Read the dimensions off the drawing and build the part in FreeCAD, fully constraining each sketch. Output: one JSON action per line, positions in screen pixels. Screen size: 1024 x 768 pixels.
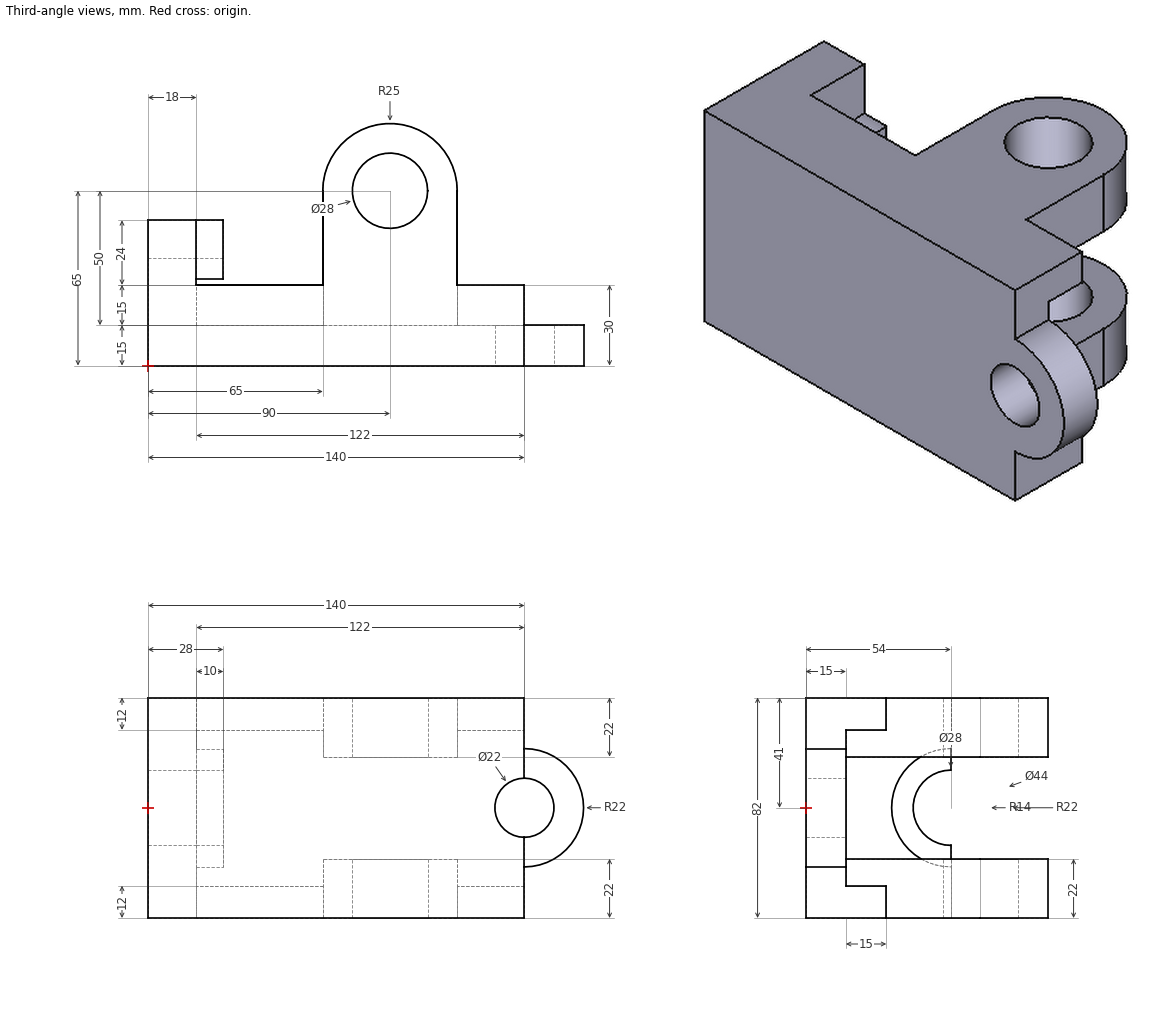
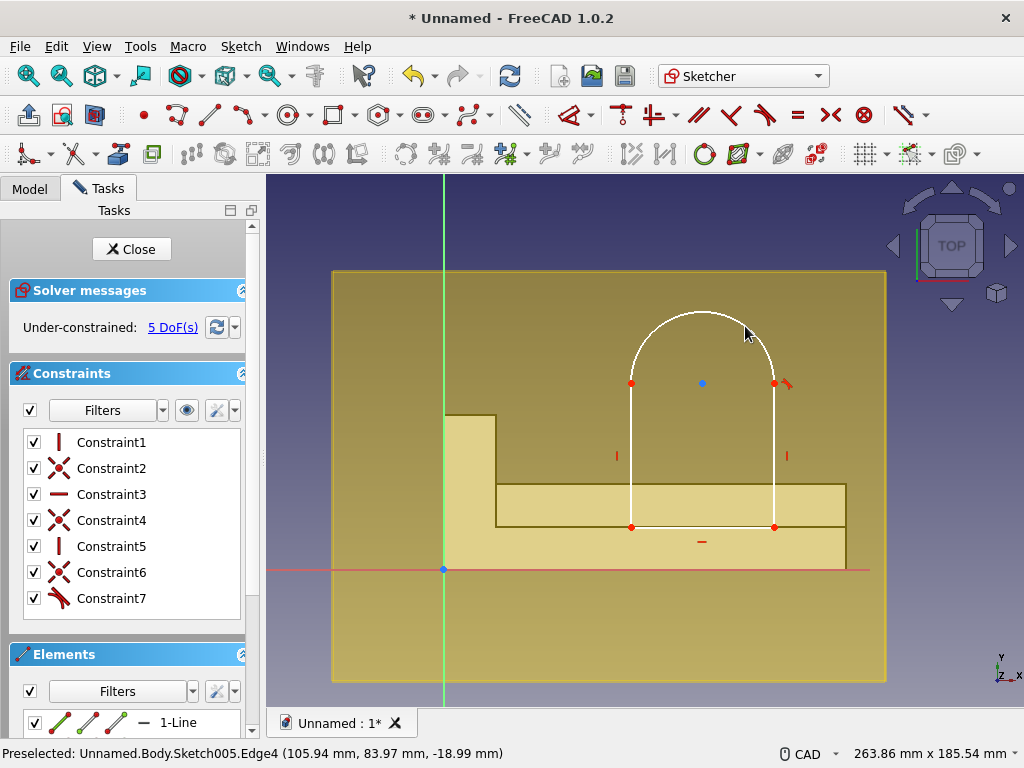
{"action": "left_click", "coordinate": [631, 485]}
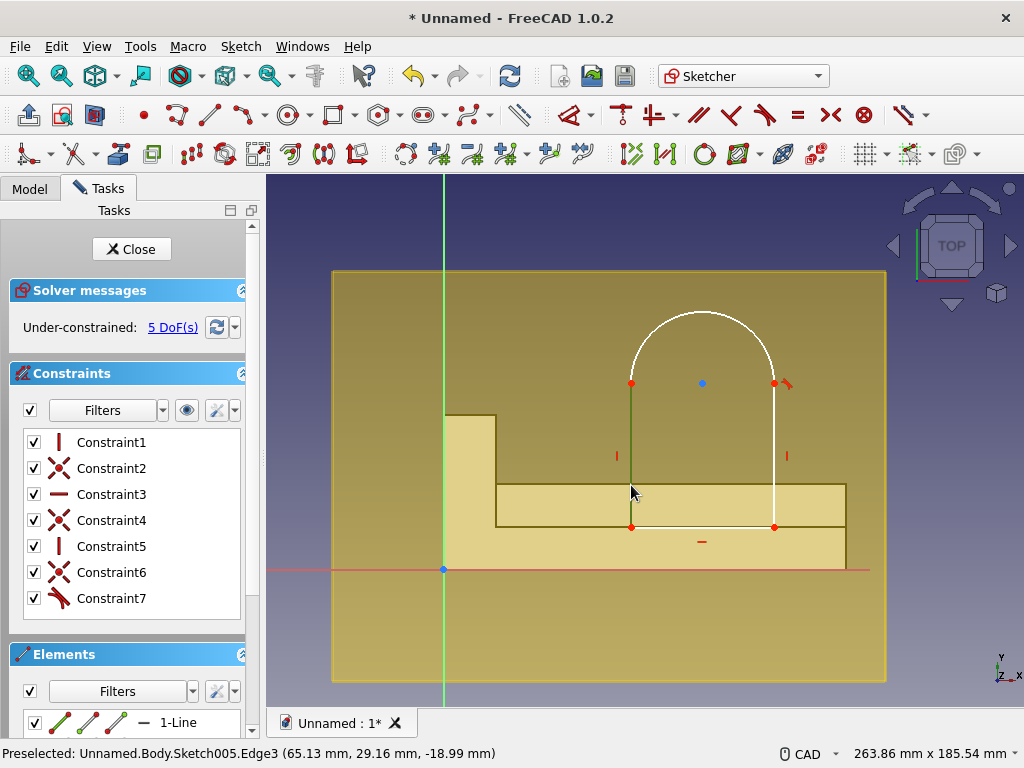
{"action": "left_click", "coordinate": [744, 326]}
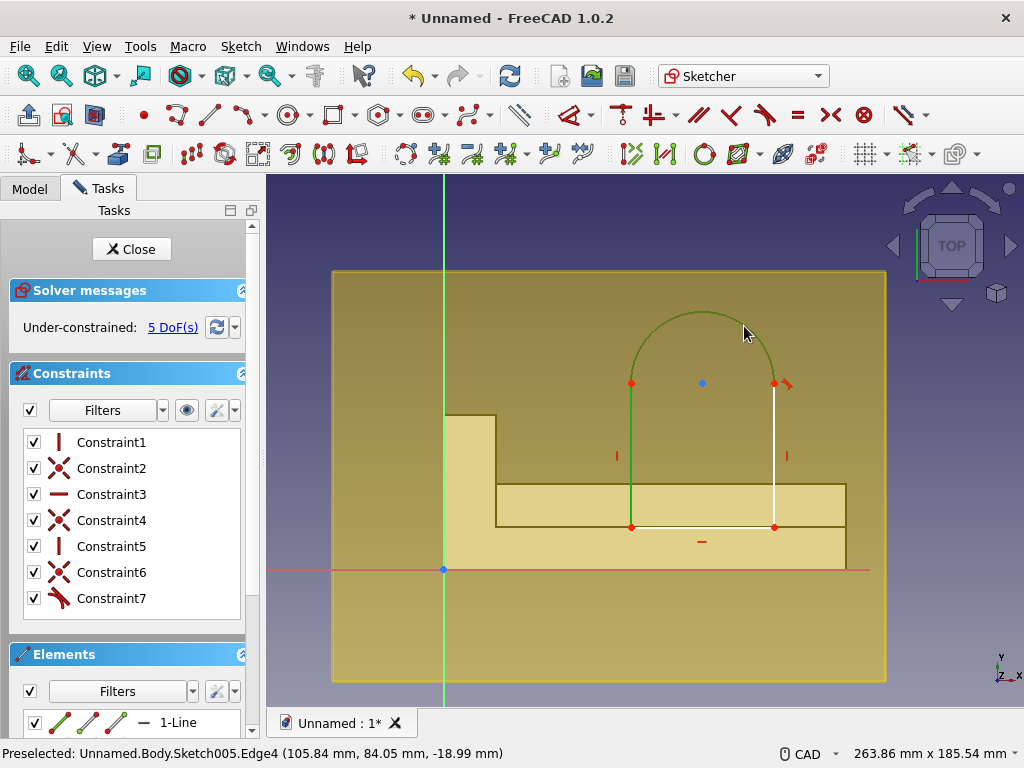
{"action": "key", "text": "t"}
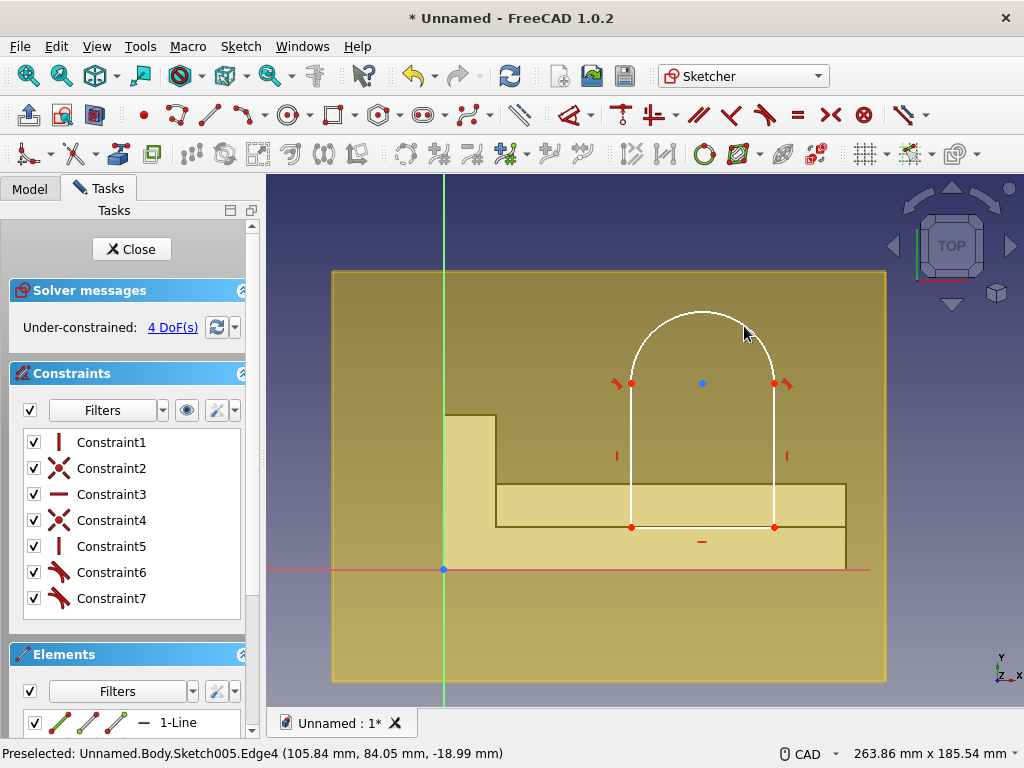
{"action": "key", "text": "d"}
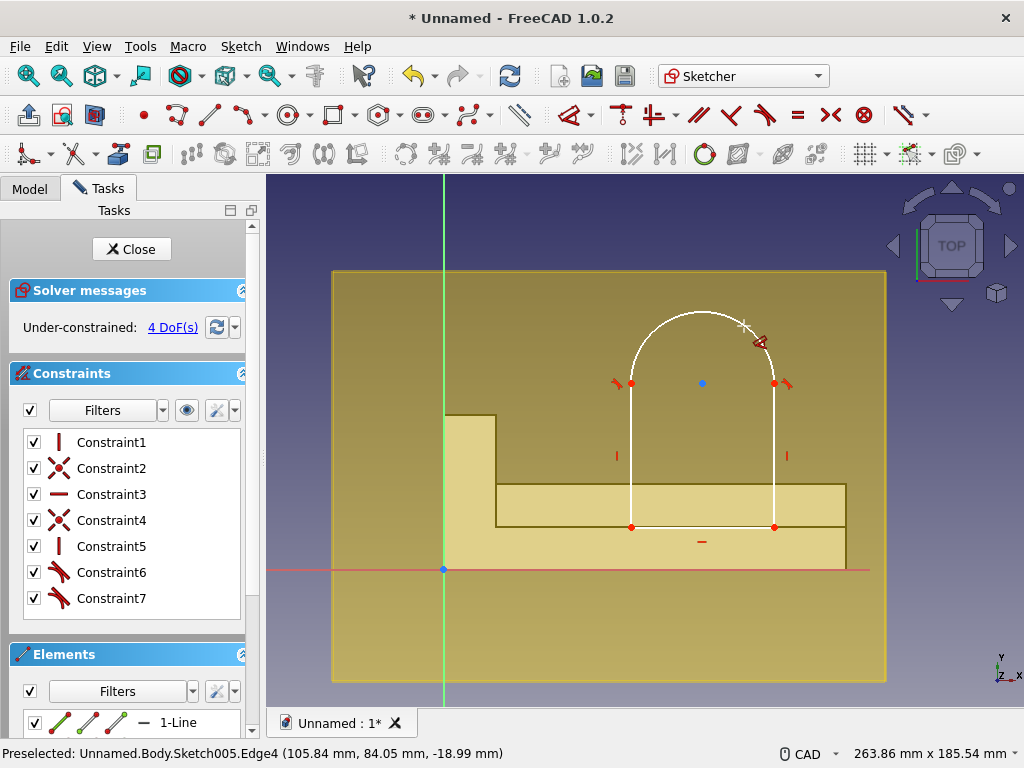
{"action": "left_click", "coordinate": [745, 326]}
{"action": "left_click", "coordinate": [764, 300]}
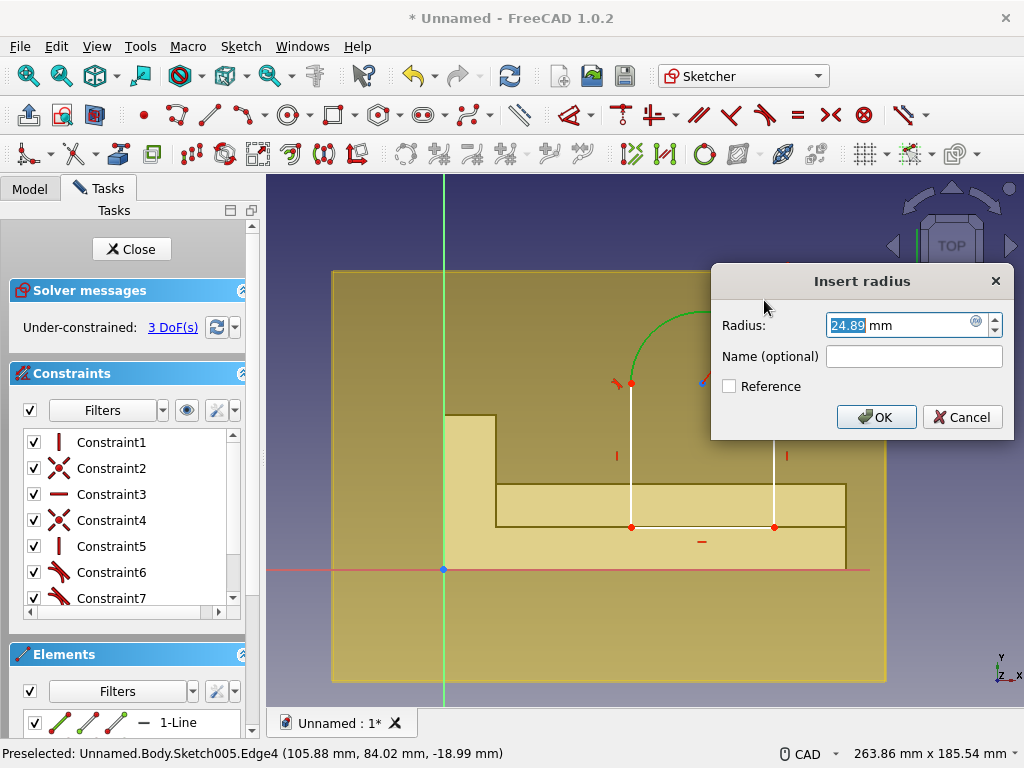
{"action": "type", "text": "25"}
{"action": "key", "text": "Return"}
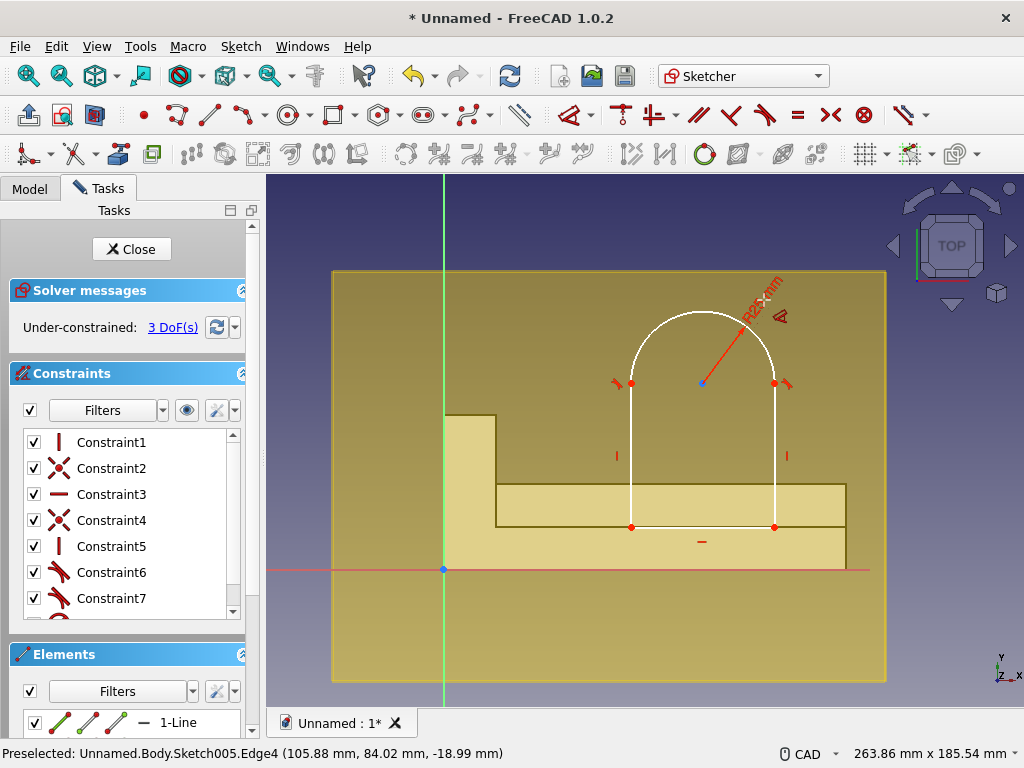
{"action": "left_click", "coordinate": [775, 427]}
{"action": "left_click", "coordinate": [809, 456]}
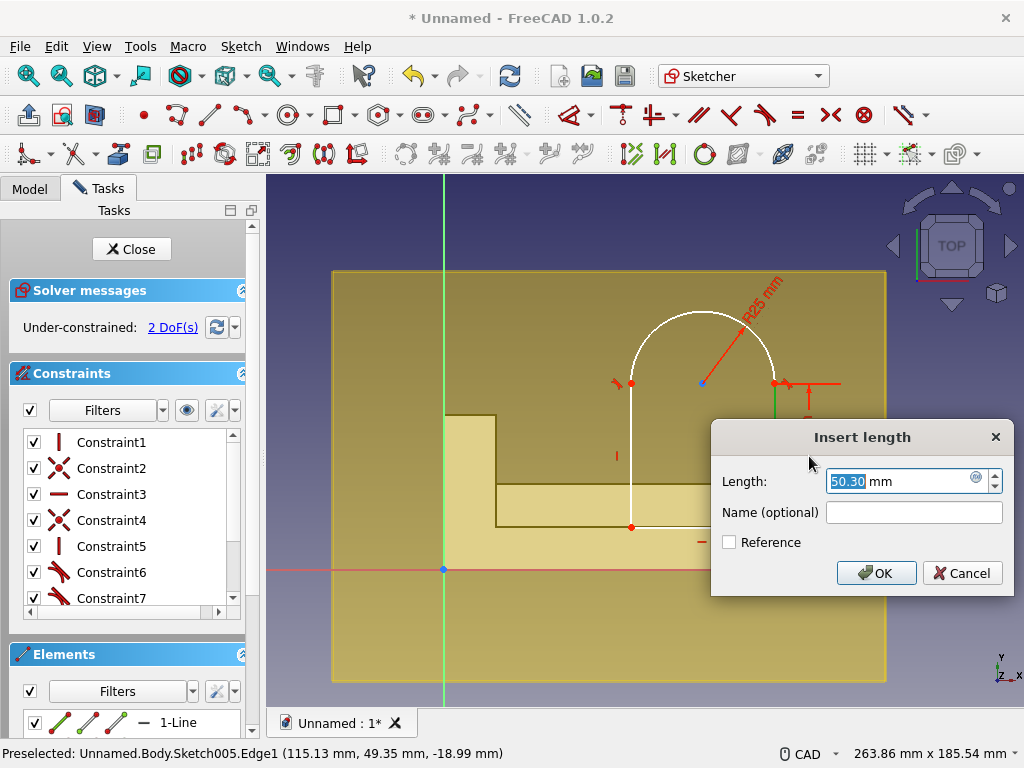
{"action": "type", "text": "50"}
{"action": "key", "text": "Return"}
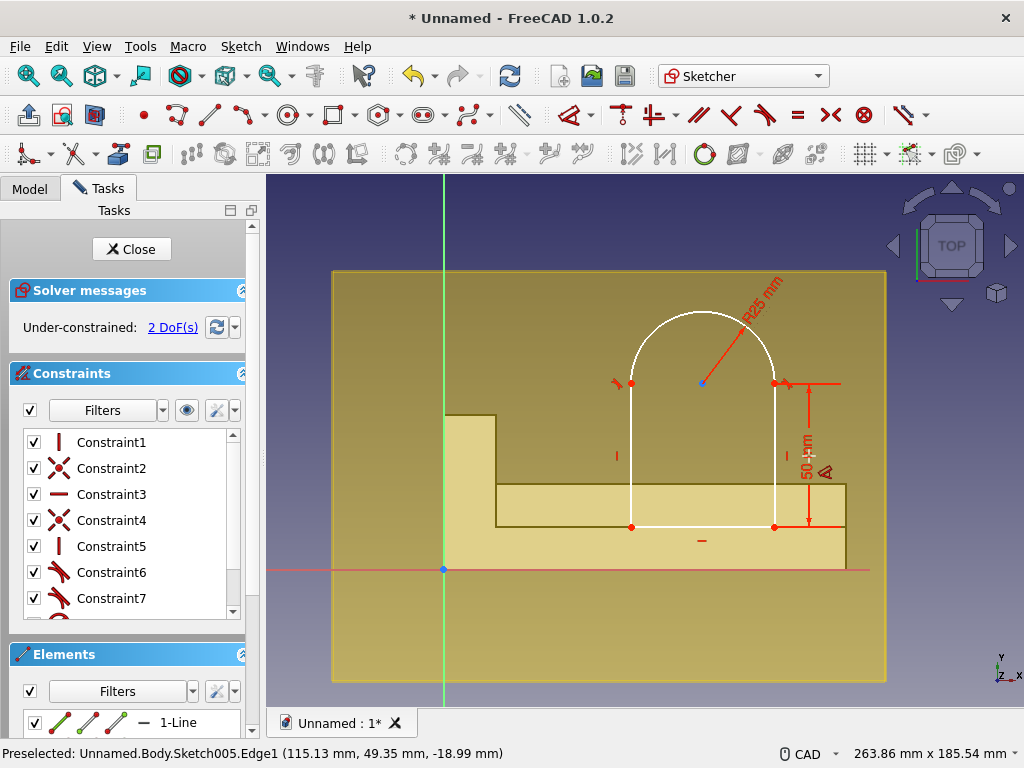
{"action": "left_click", "coordinate": [775, 384]}
{"action": "left_click", "coordinate": [809, 477]}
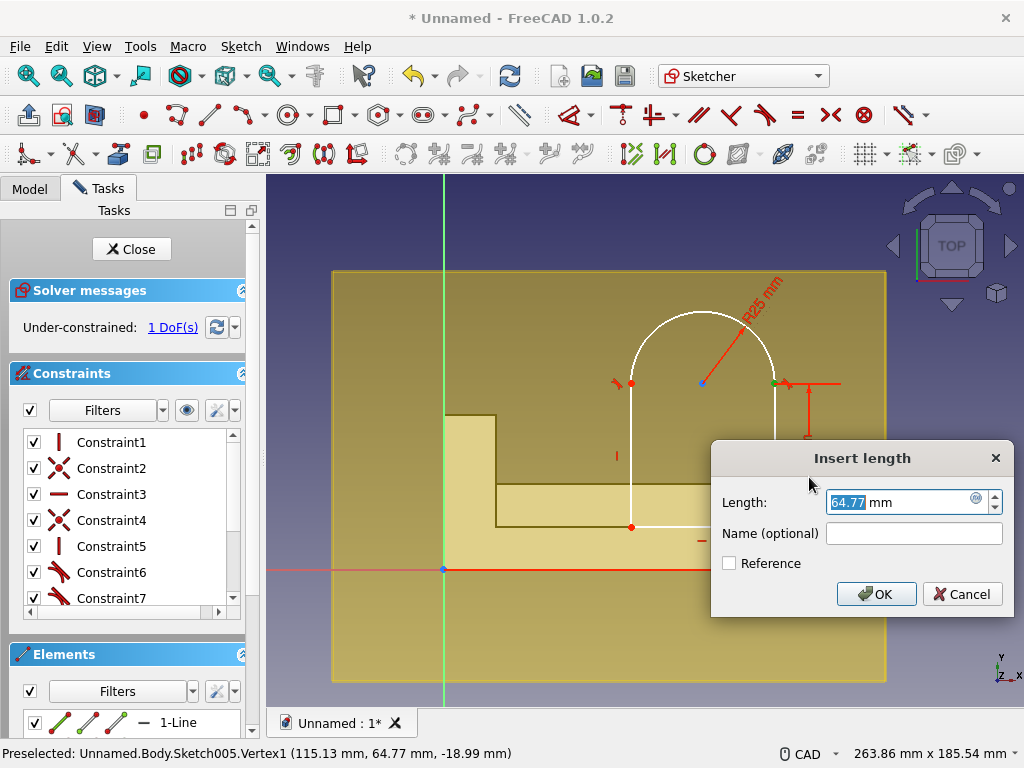
{"action": "type", "text": "65"}
{"action": "key", "text": "Return"}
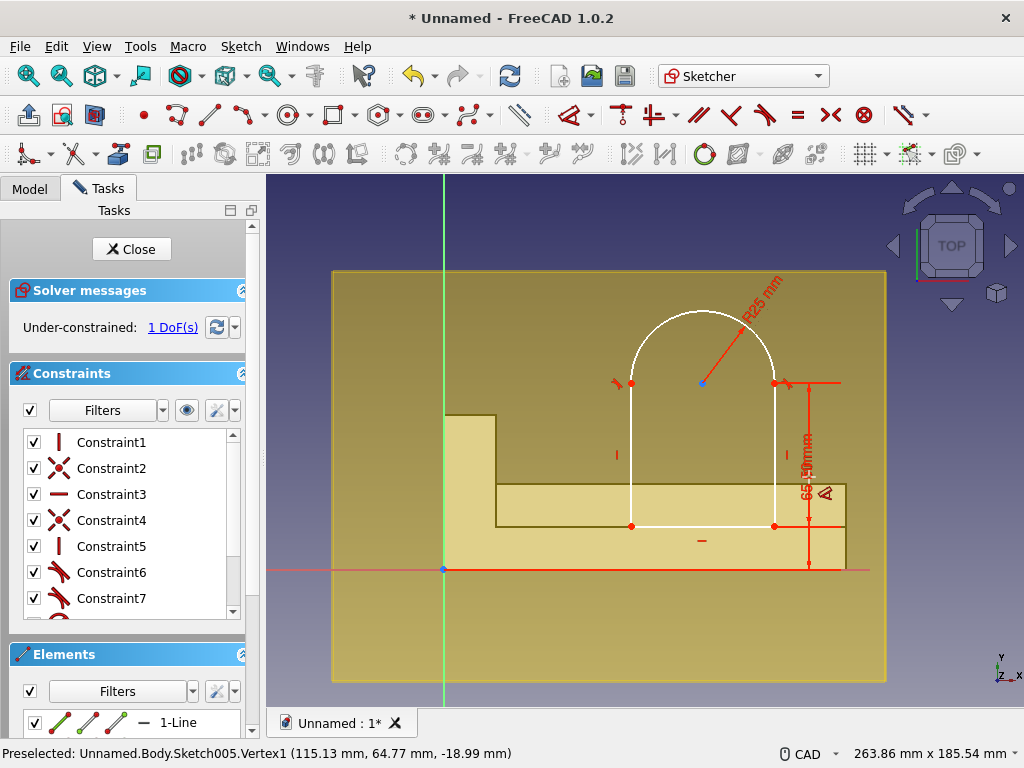
{"action": "left_click", "coordinate": [631, 527]}
{"action": "left_click", "coordinate": [537, 604]}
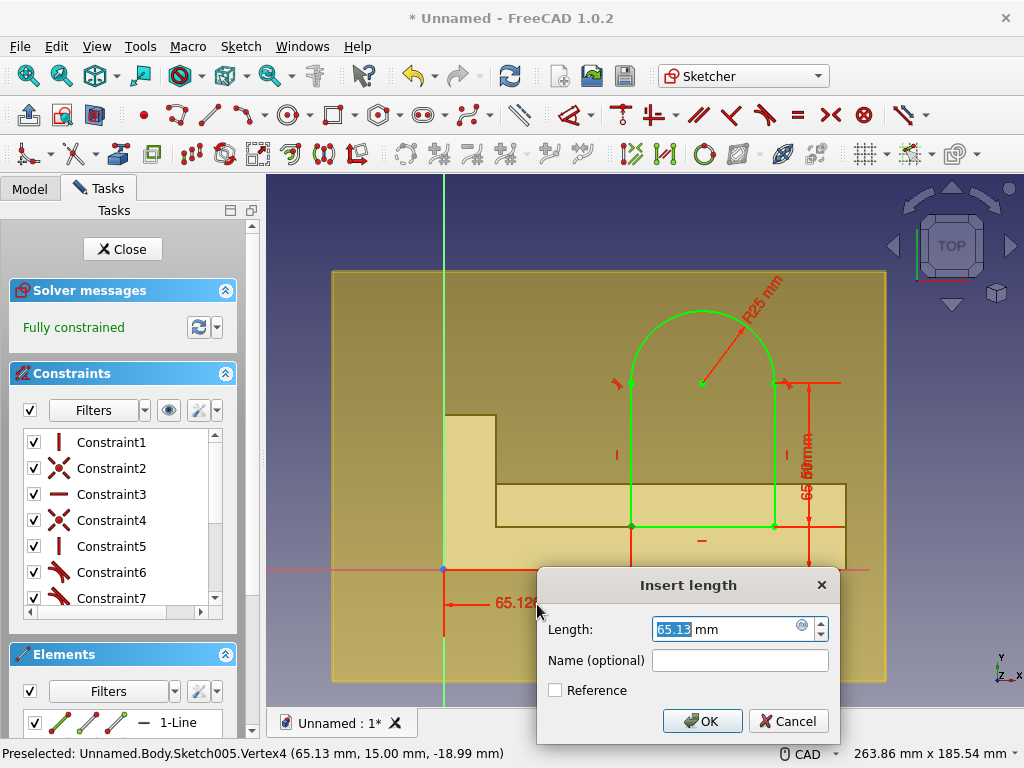
{"action": "type", "text": "65"}
{"action": "key", "text": "Return"}
{"action": "key", "text": "Escape"}